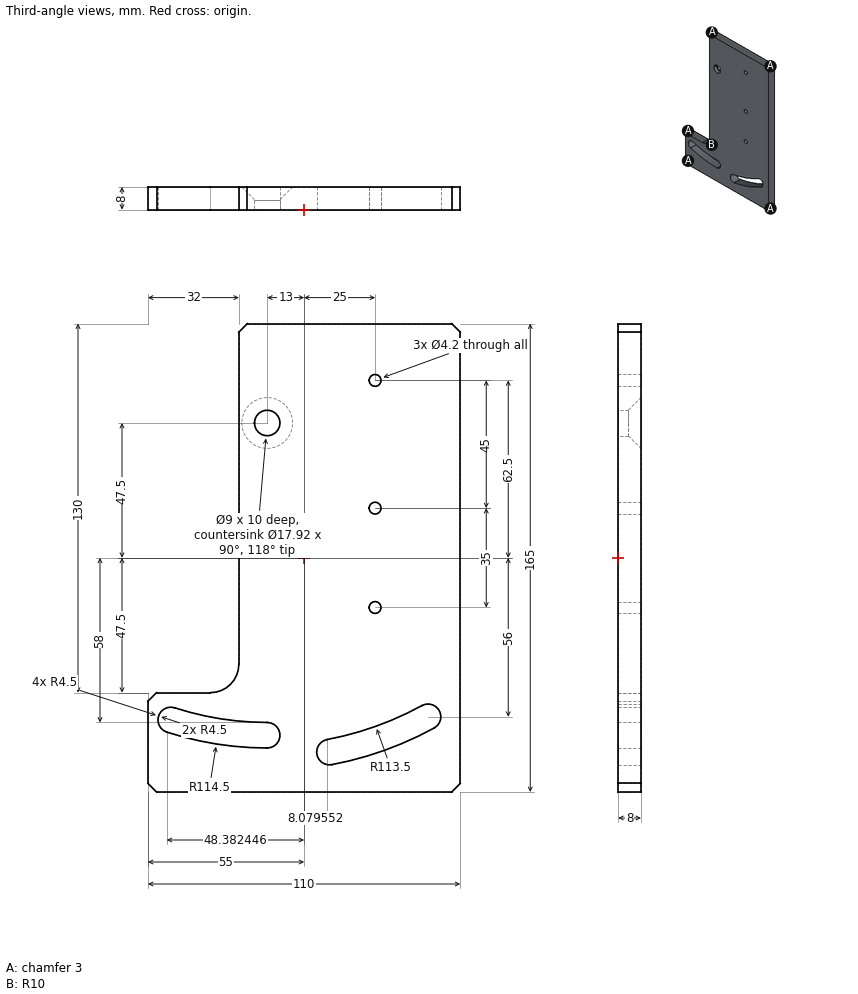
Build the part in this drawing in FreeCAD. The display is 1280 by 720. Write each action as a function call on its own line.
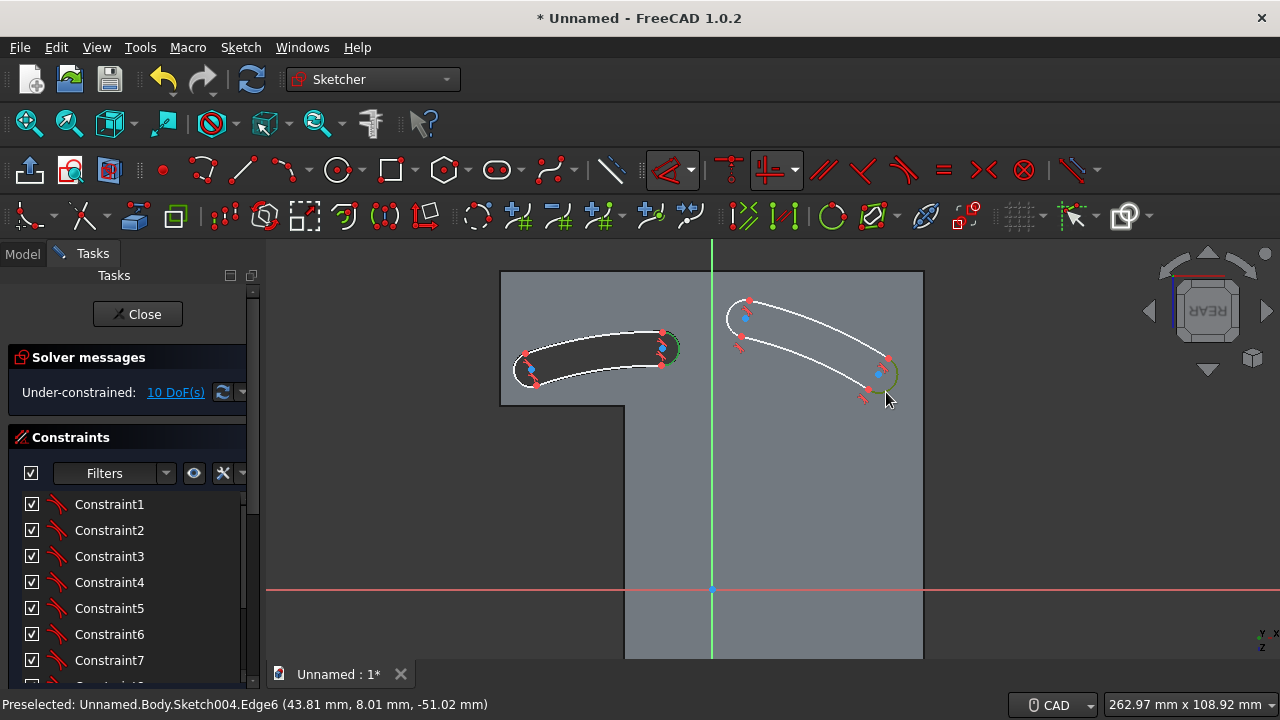
click(944, 170)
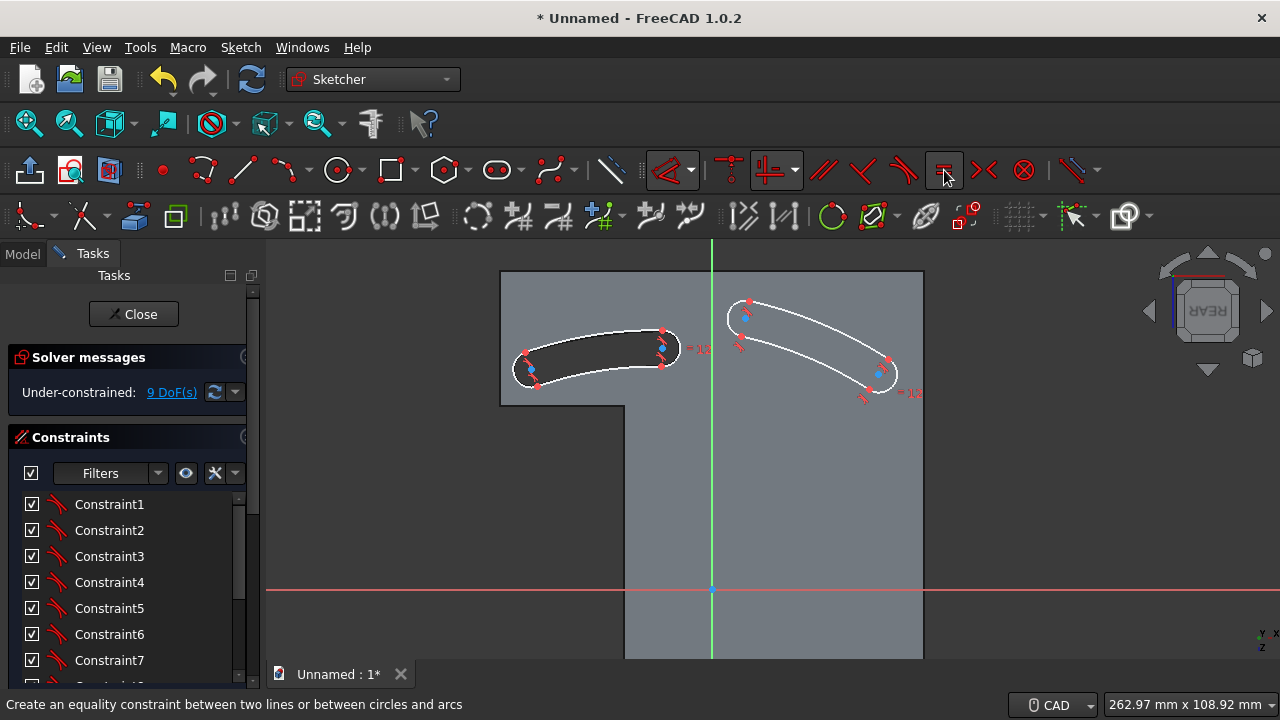
scroll(677, 359, up, 5)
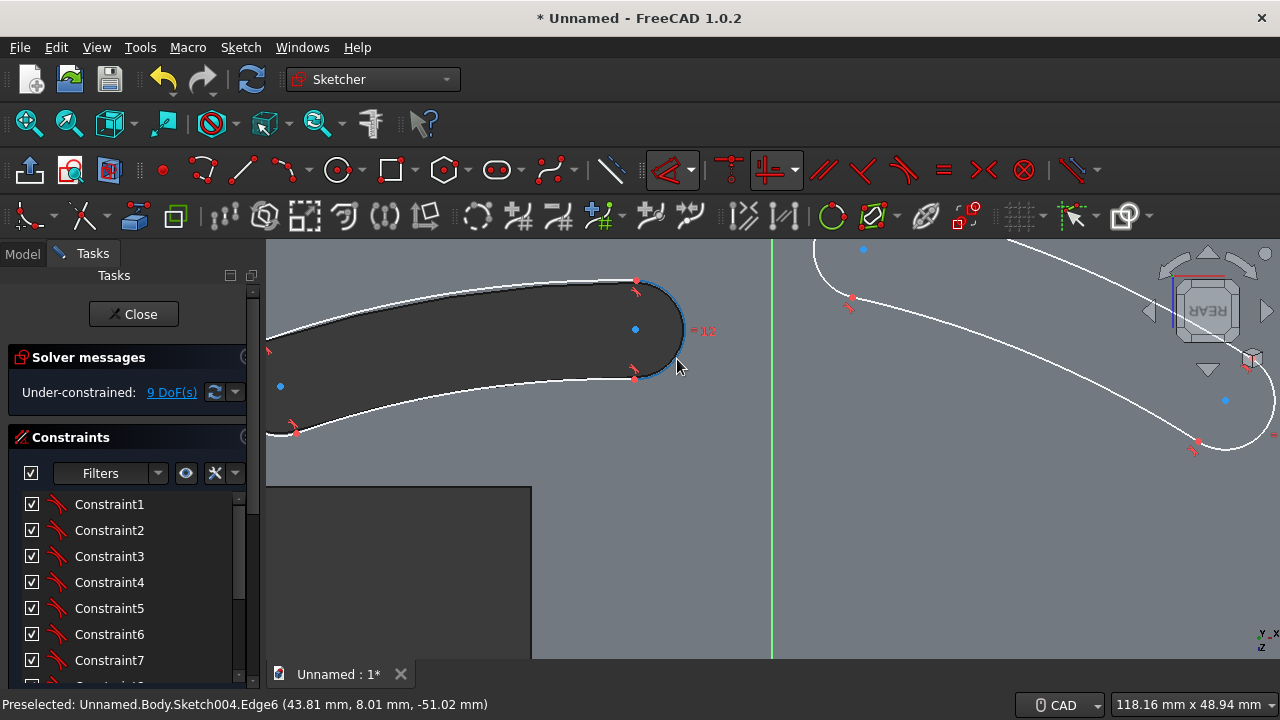
click(675, 360)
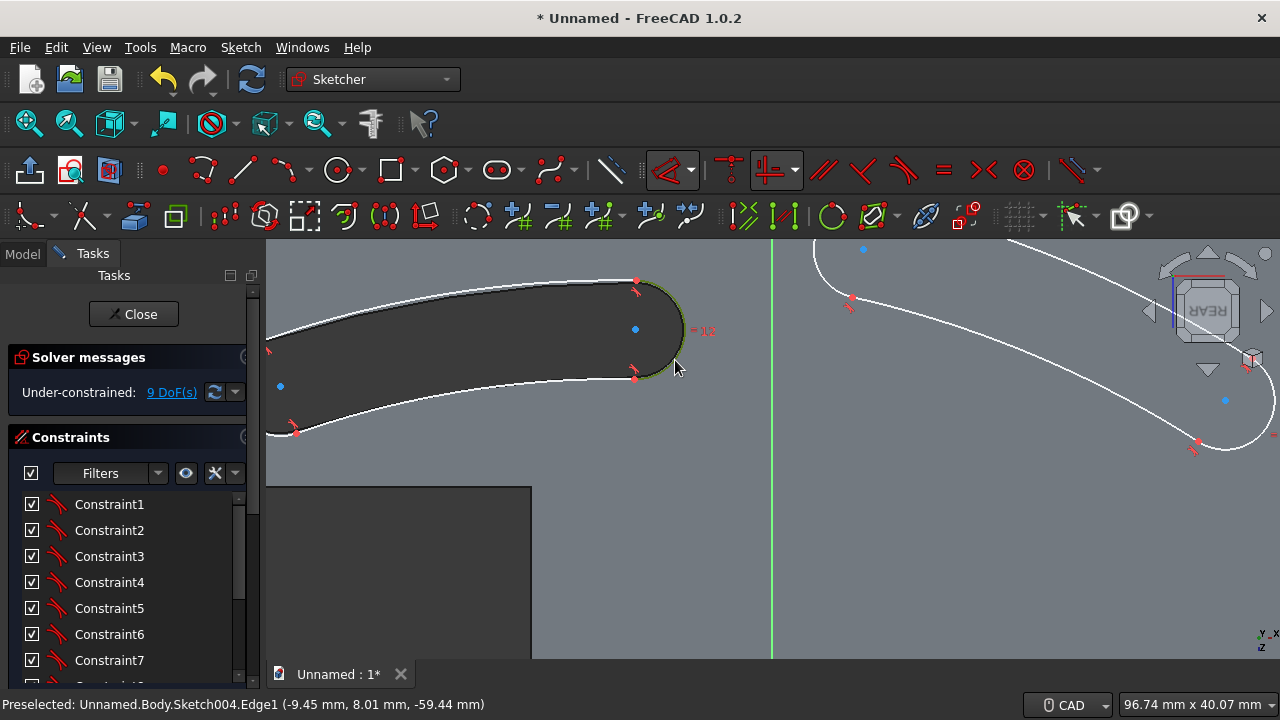
click(694, 170)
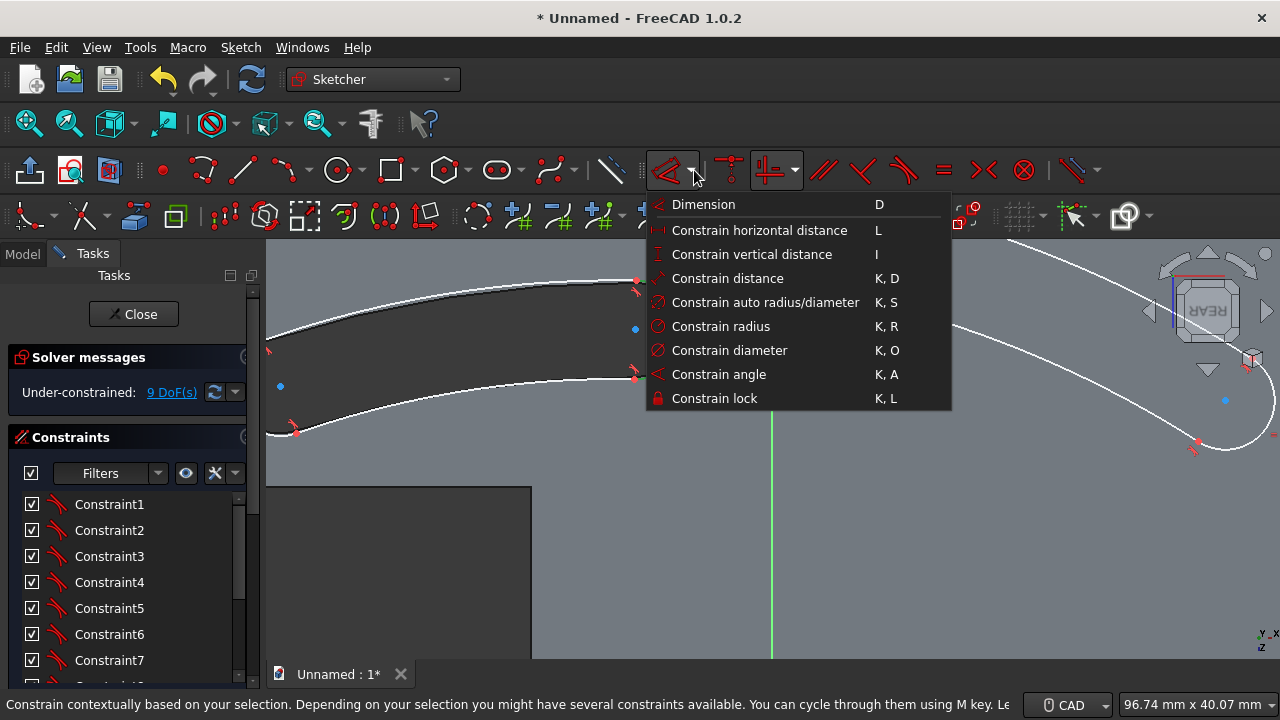
click(799, 326)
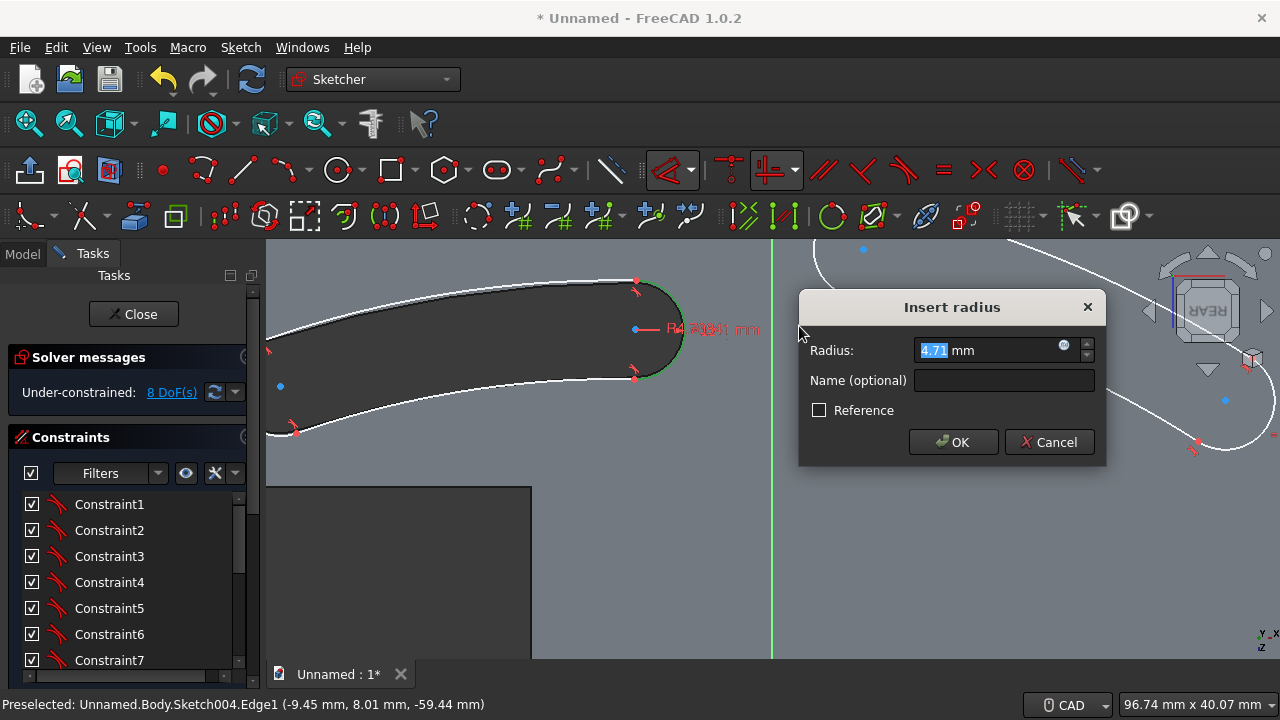
text(4.5)
key(Return)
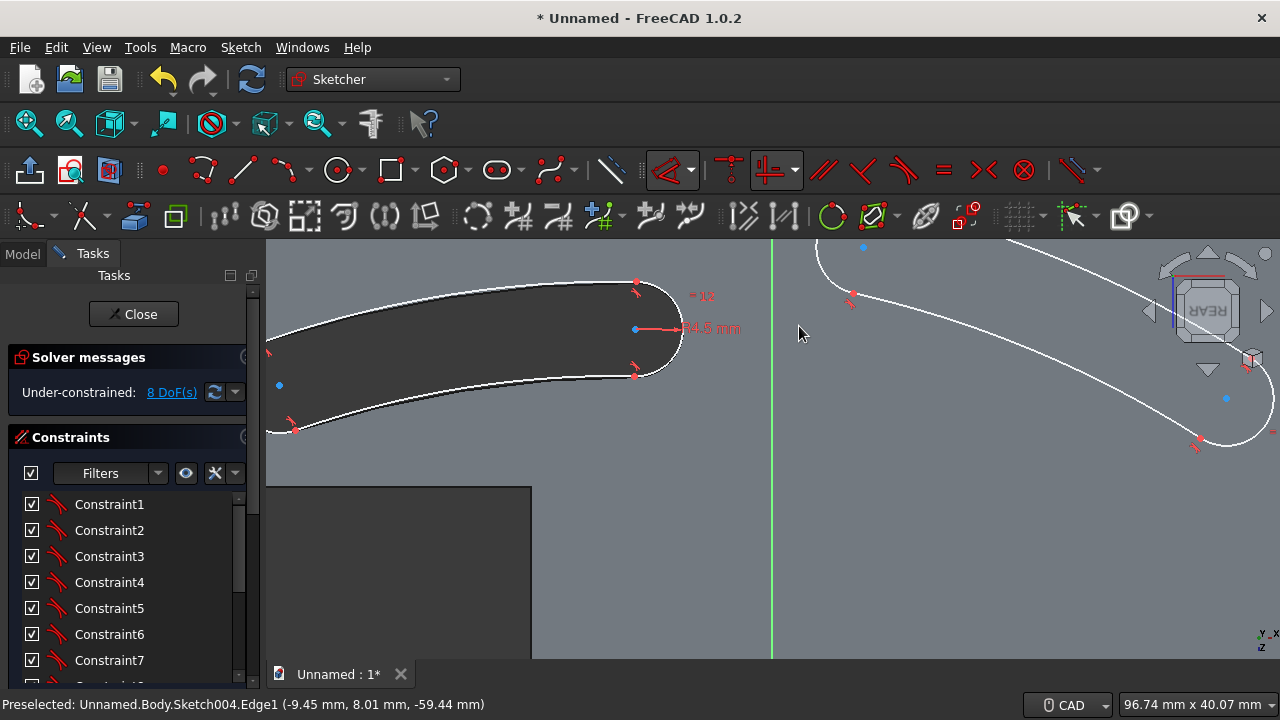
click(523, 286)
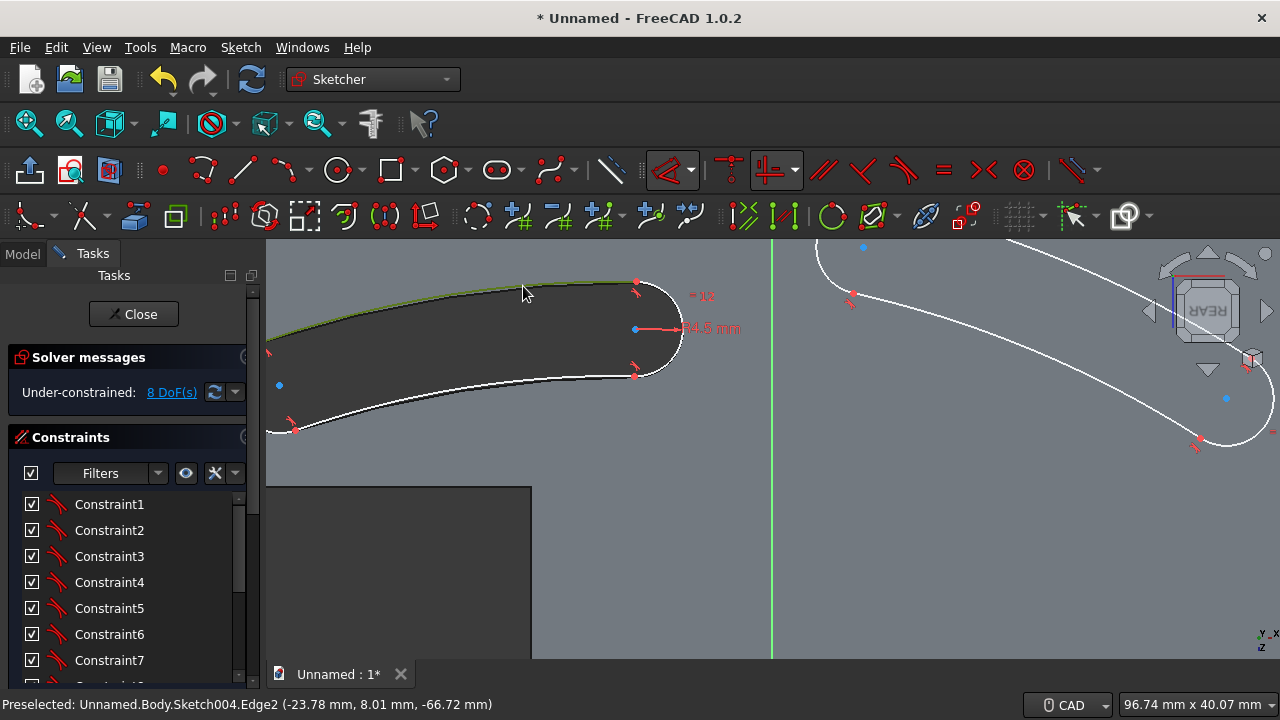
click(694, 170)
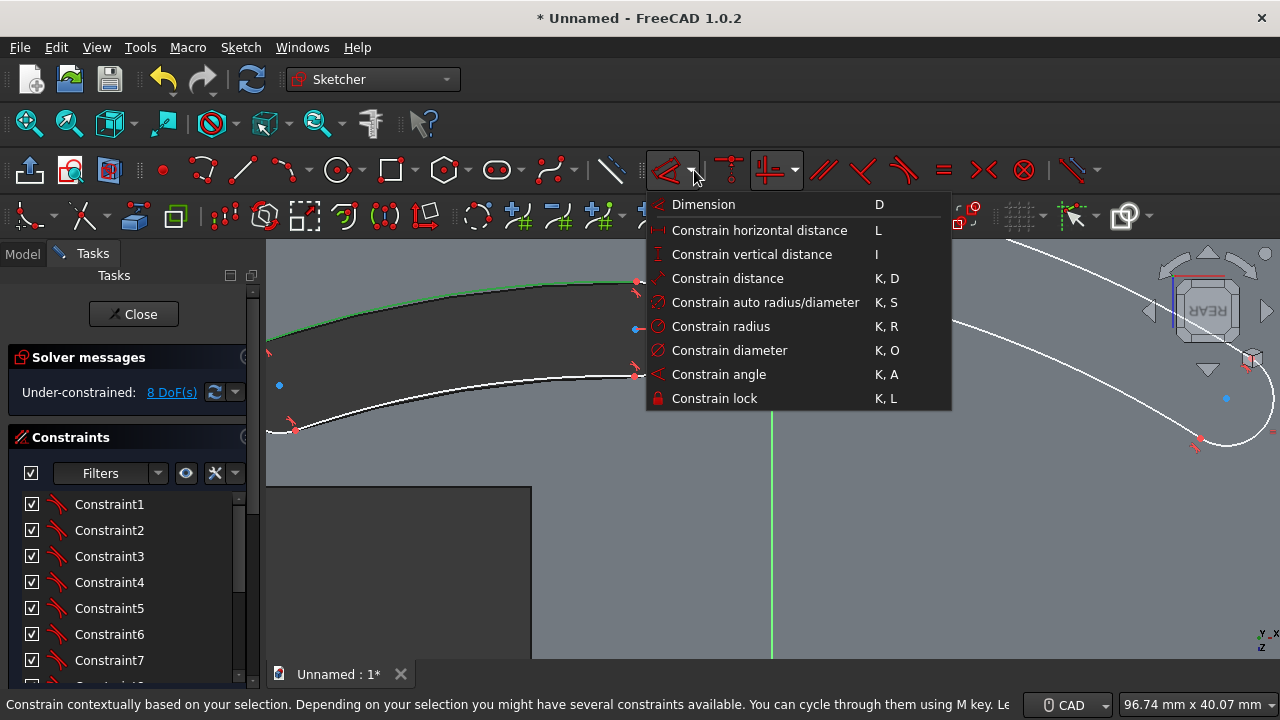
click(799, 326)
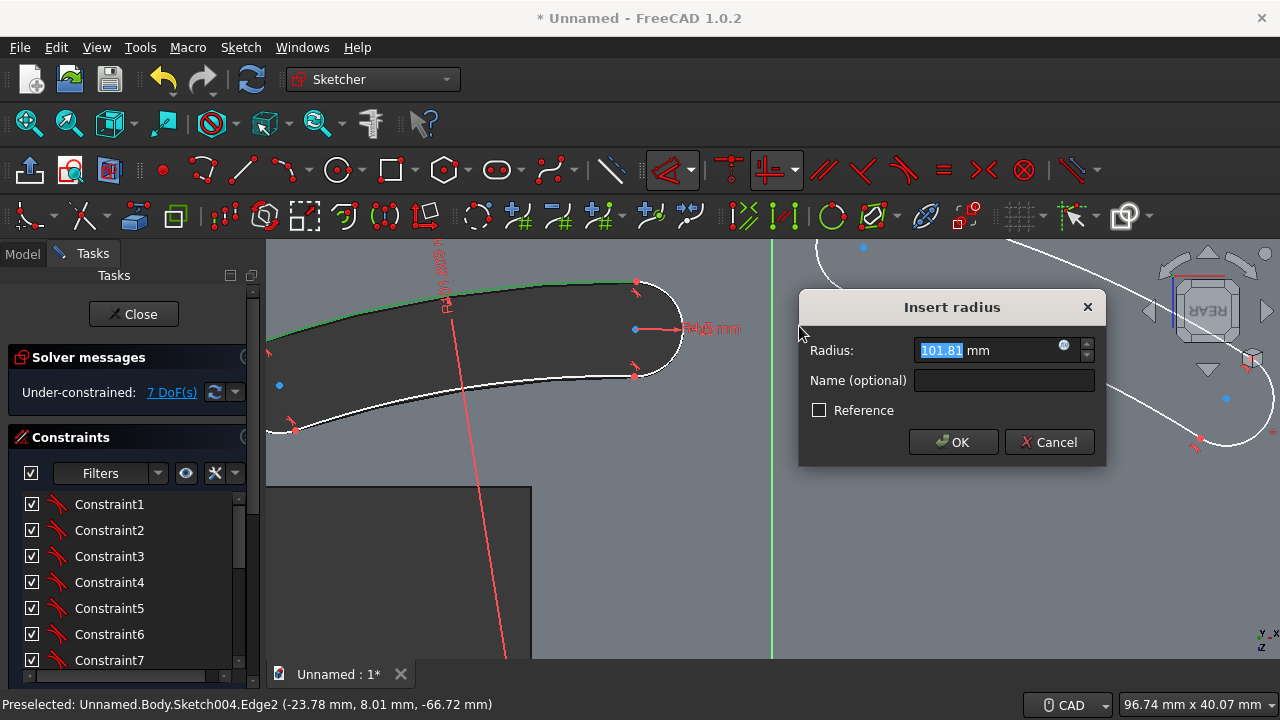
text(114.5)
key(Return)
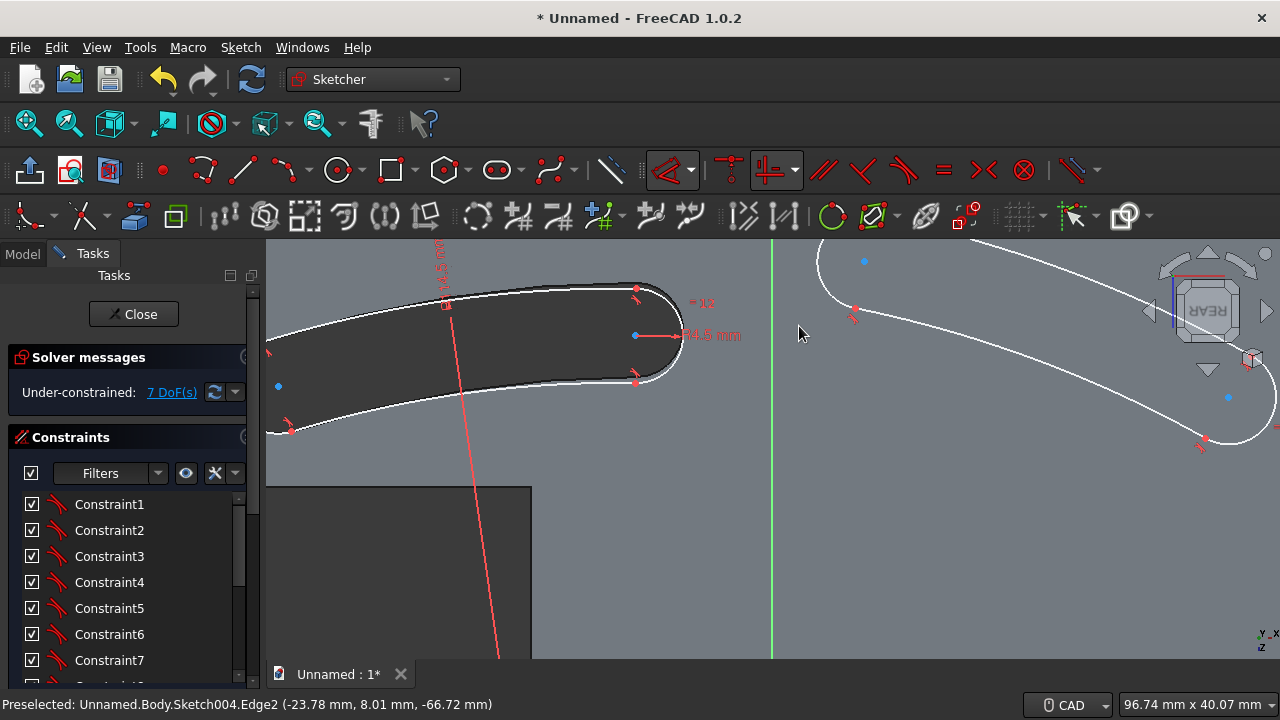
click(1105, 388)